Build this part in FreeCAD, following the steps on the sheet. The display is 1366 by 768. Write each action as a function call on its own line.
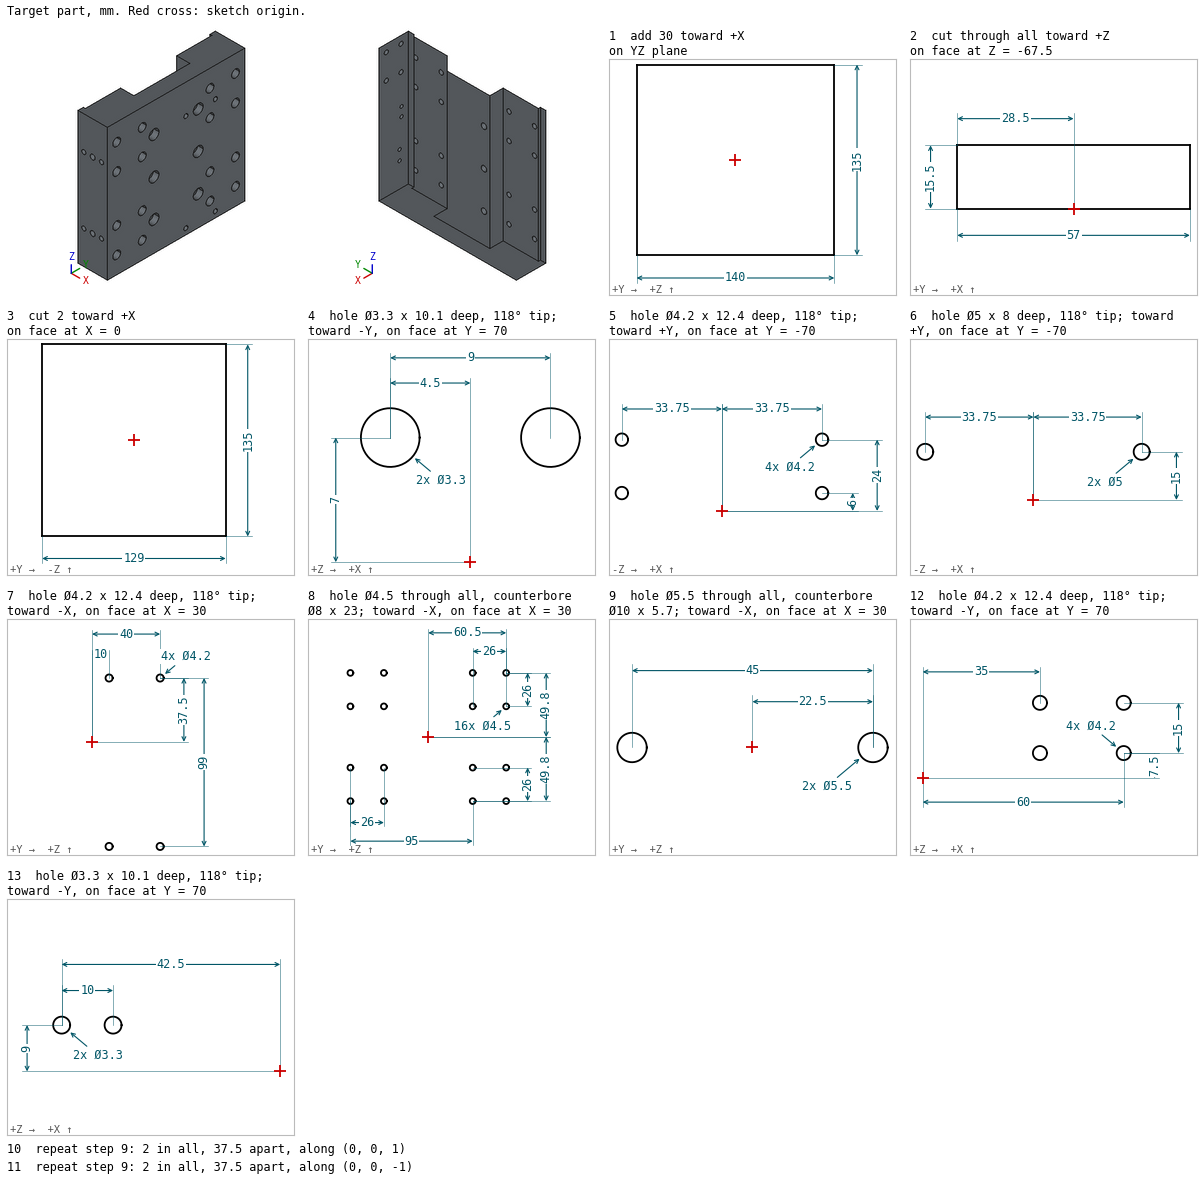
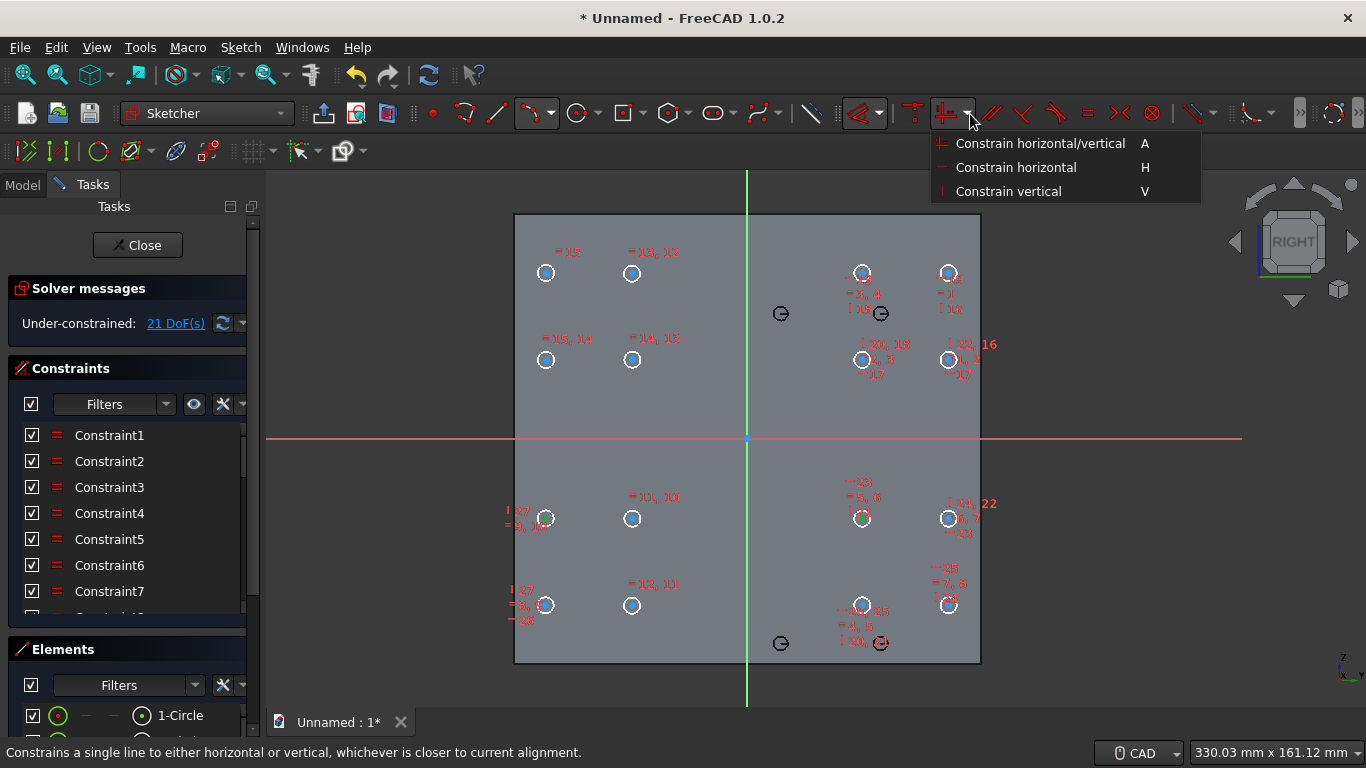
click(1066, 167)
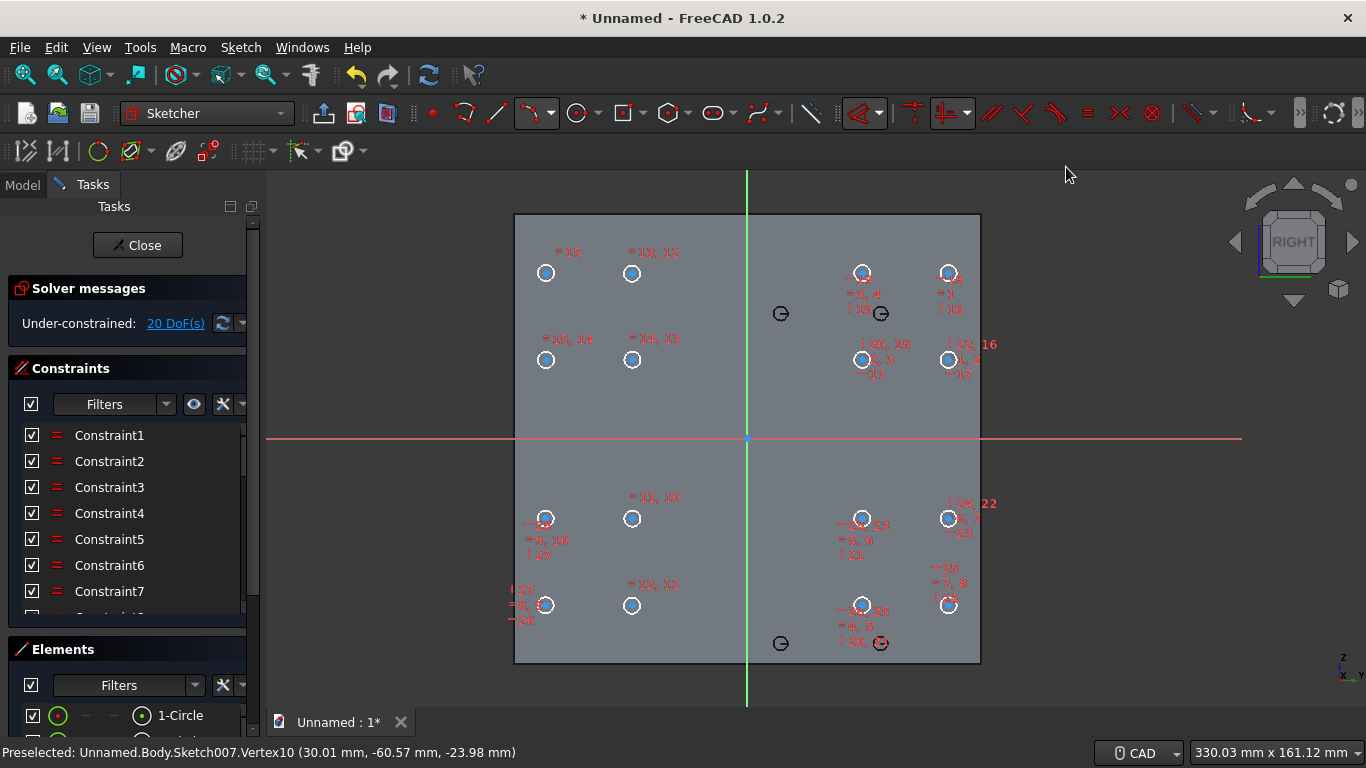
scroll(546, 519, up, 4)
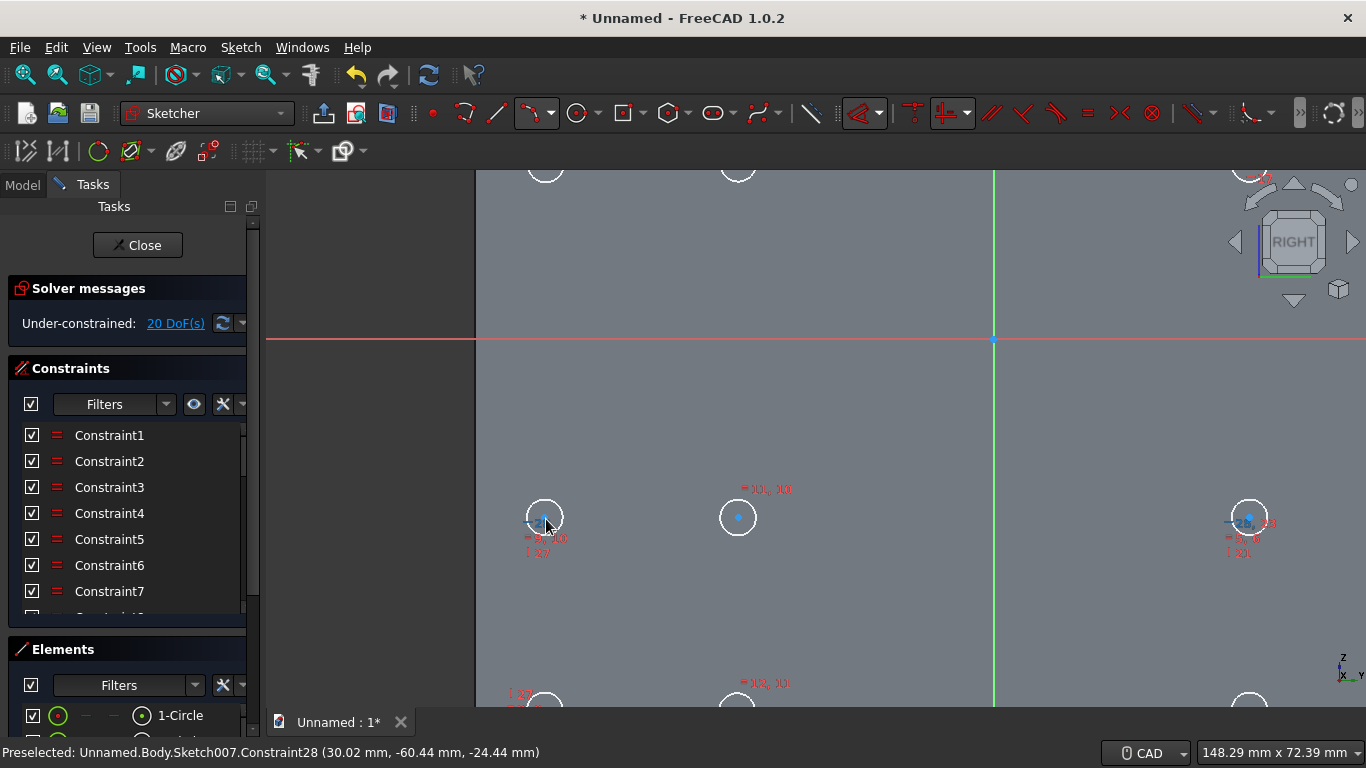
click(543, 515)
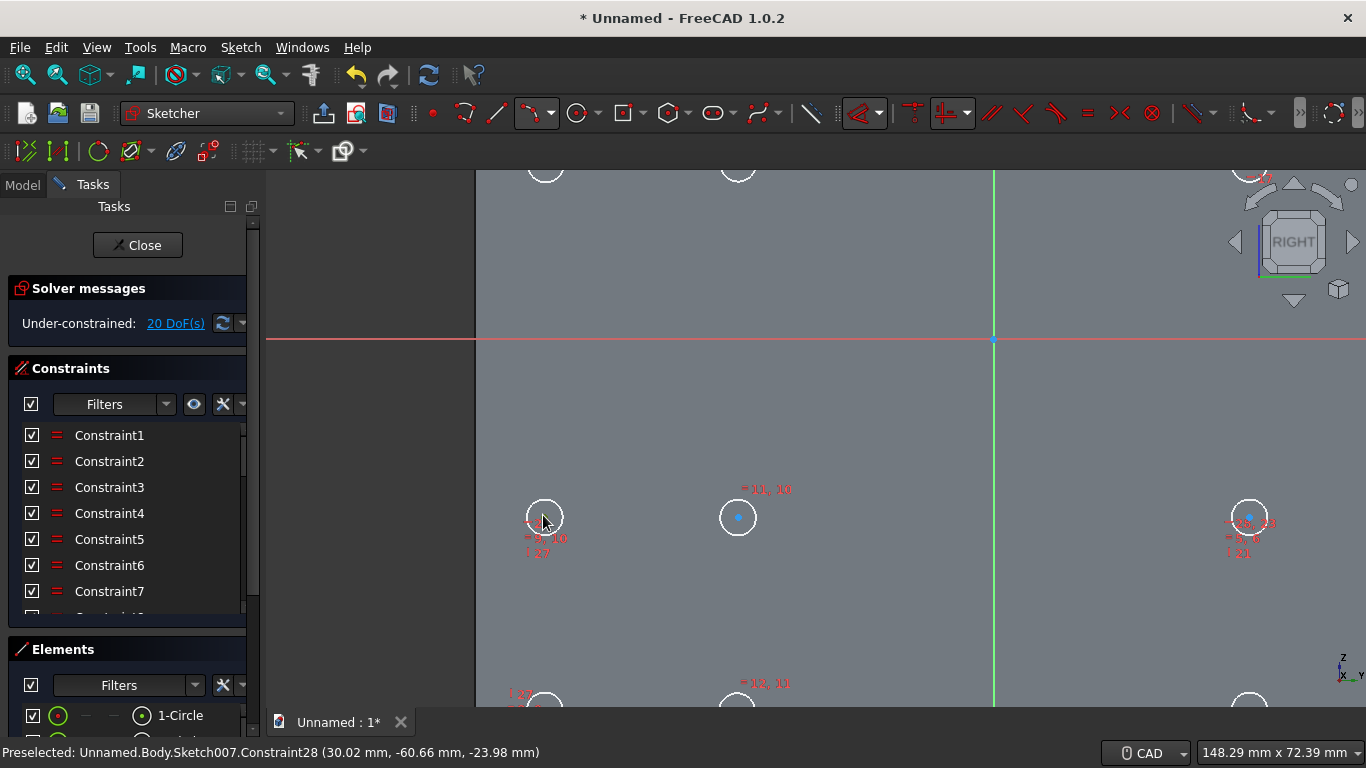
click(738, 518)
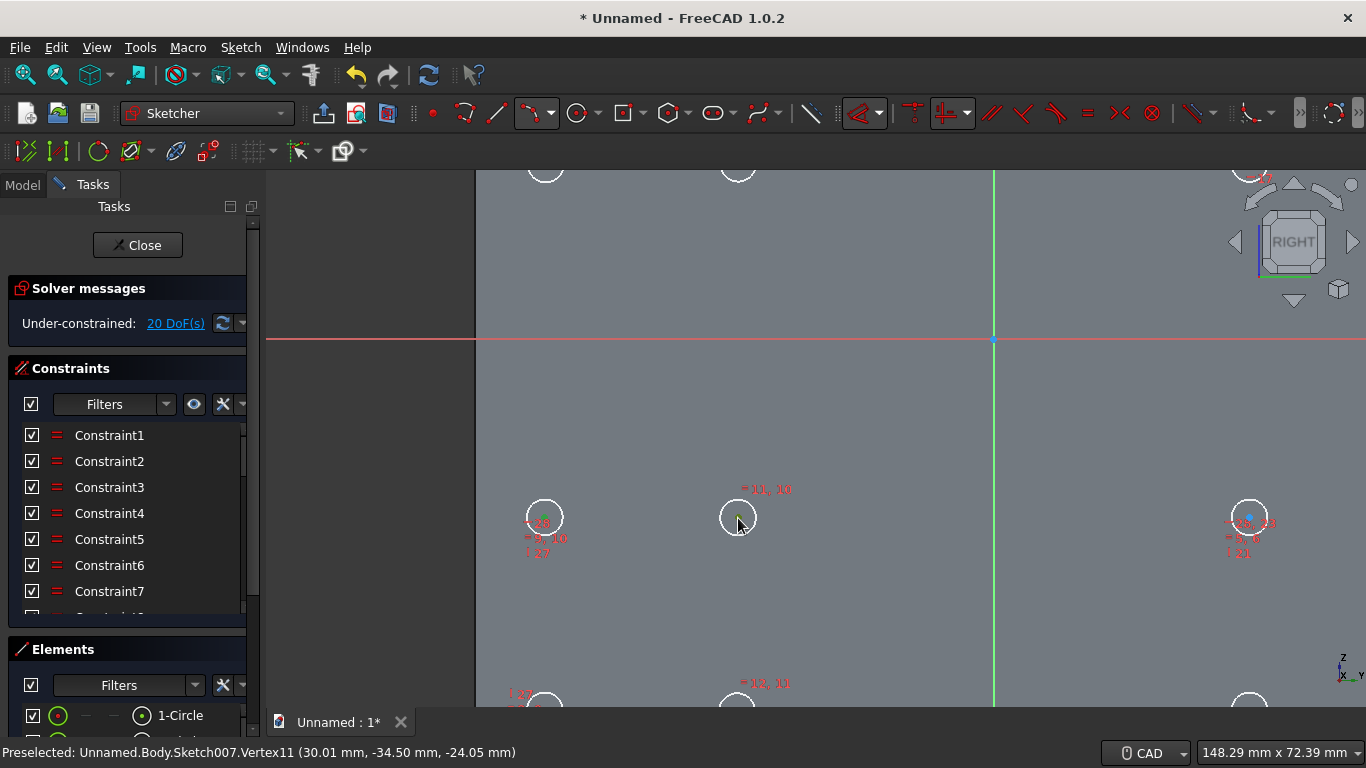
click(970, 114)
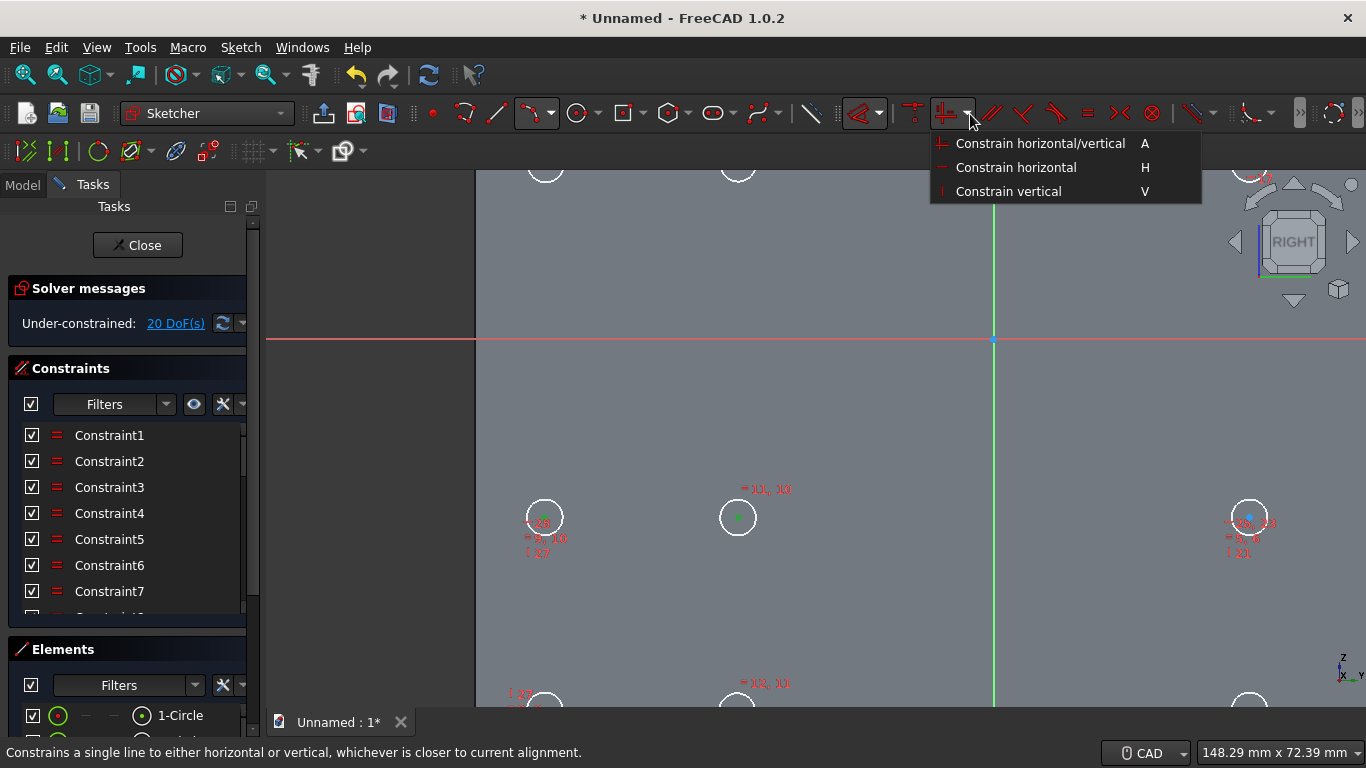
click(1066, 167)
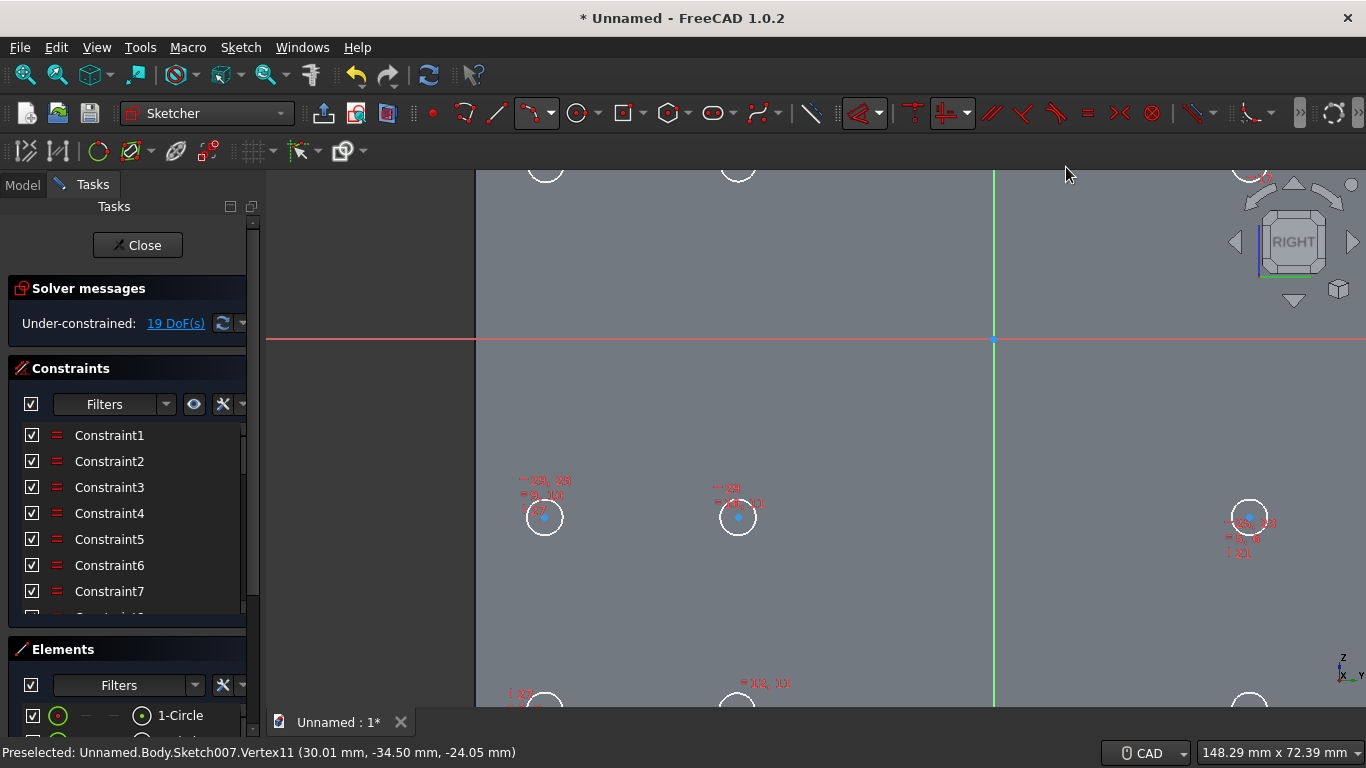
click(738, 517)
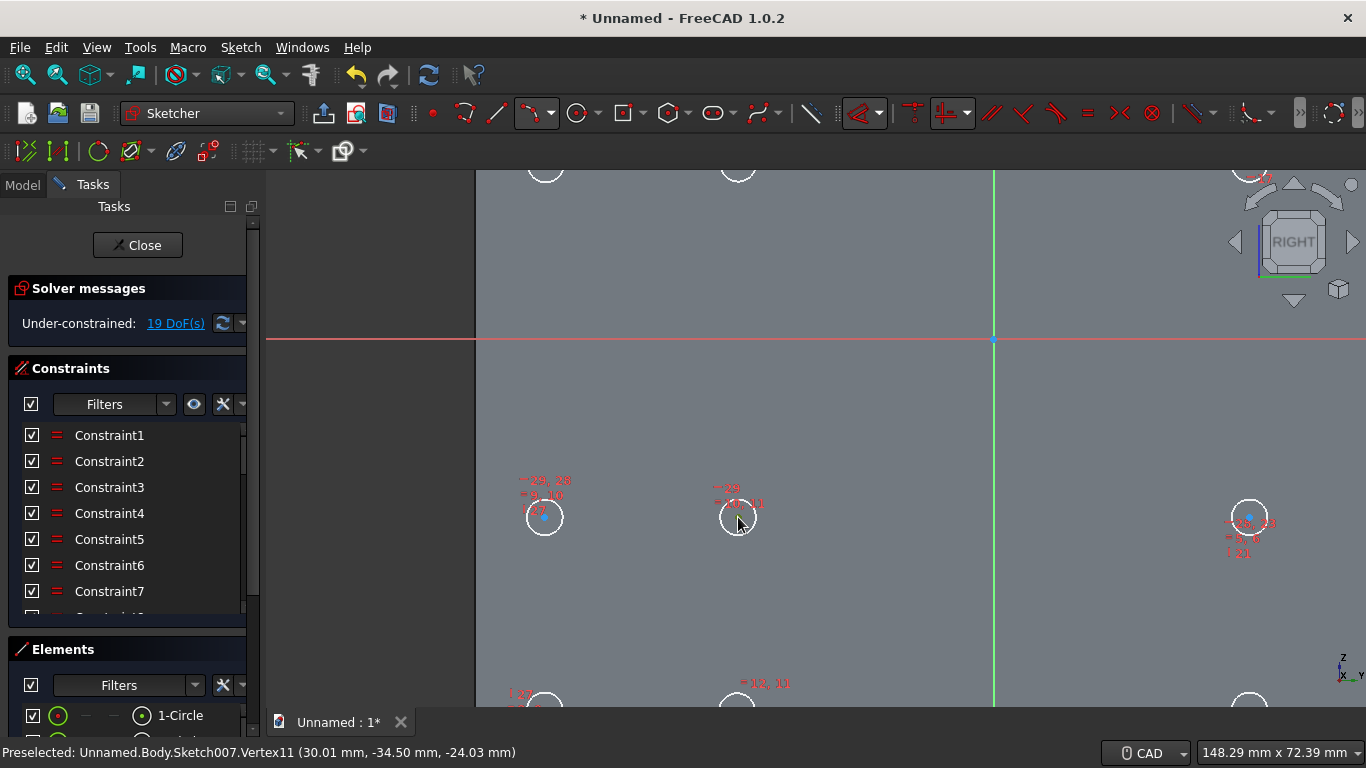
scroll(546, 520, down, 4)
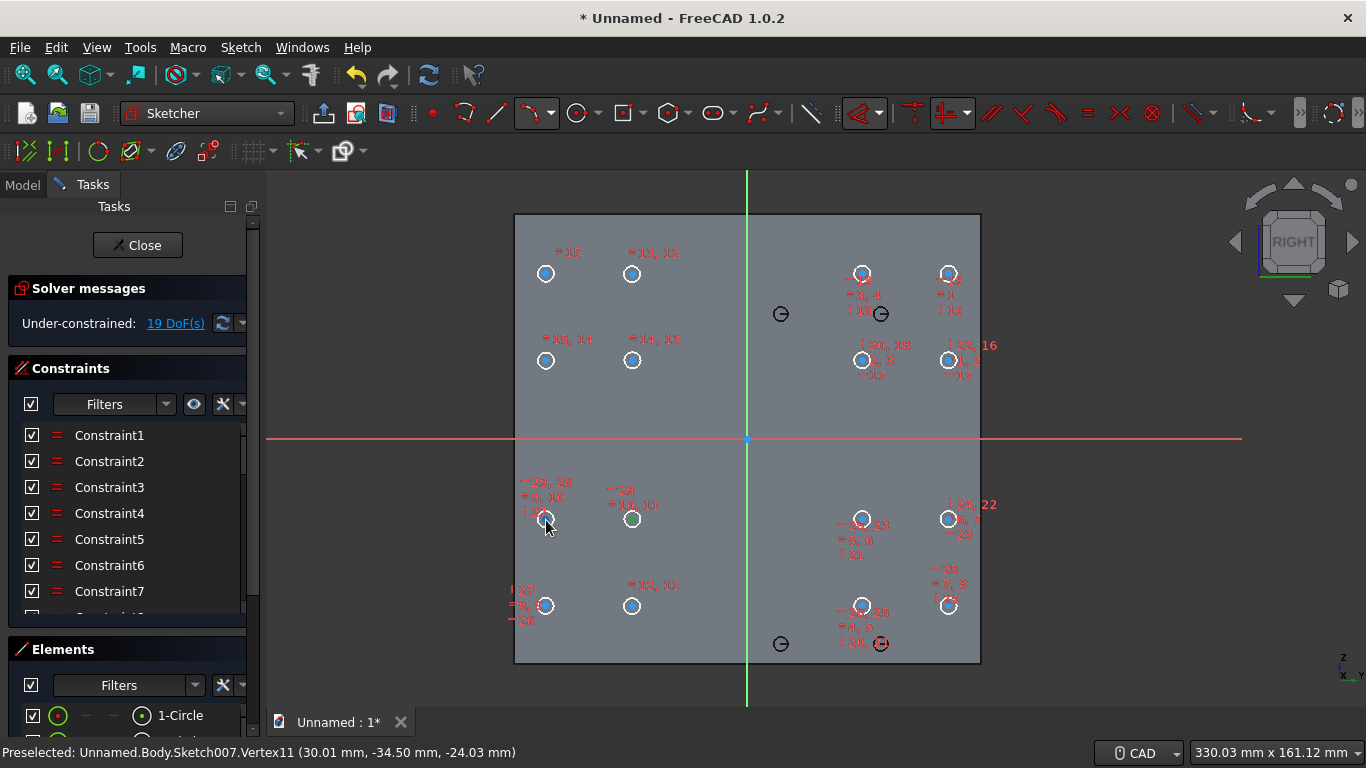
click(632, 606)